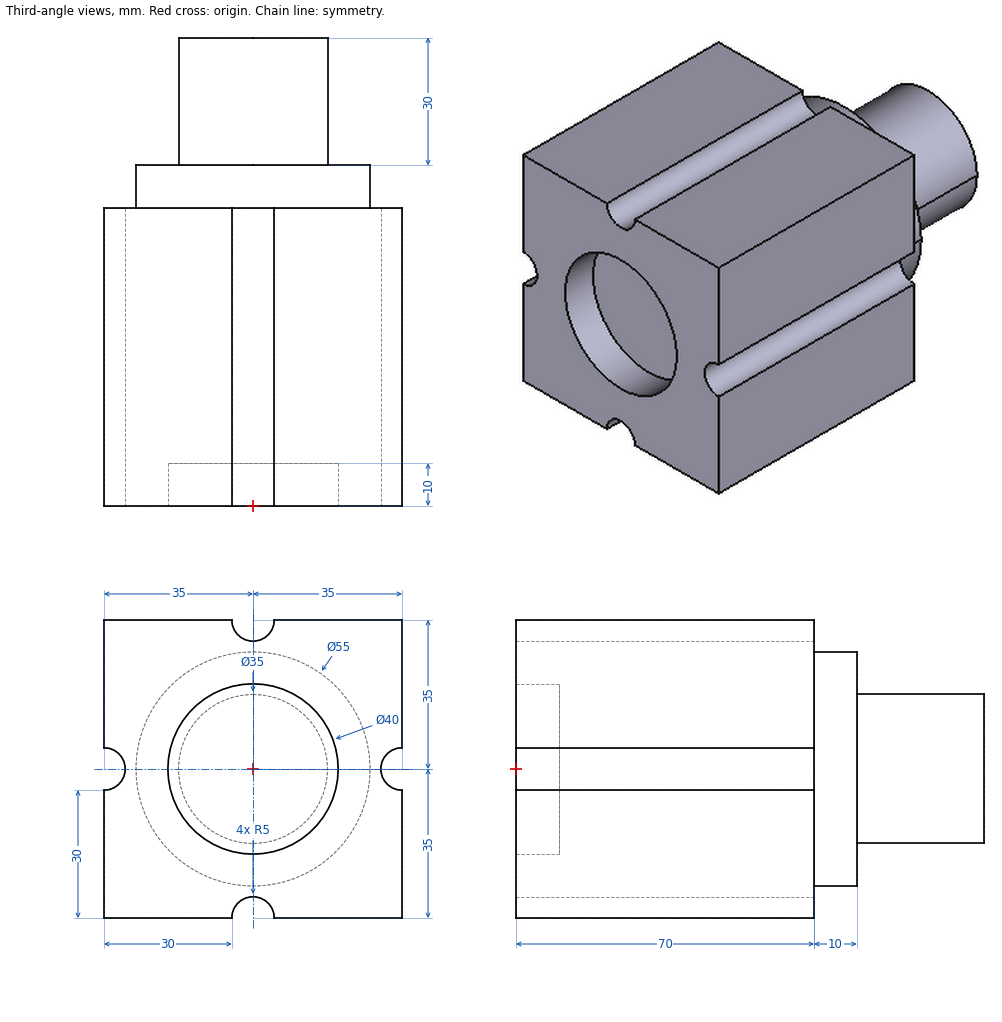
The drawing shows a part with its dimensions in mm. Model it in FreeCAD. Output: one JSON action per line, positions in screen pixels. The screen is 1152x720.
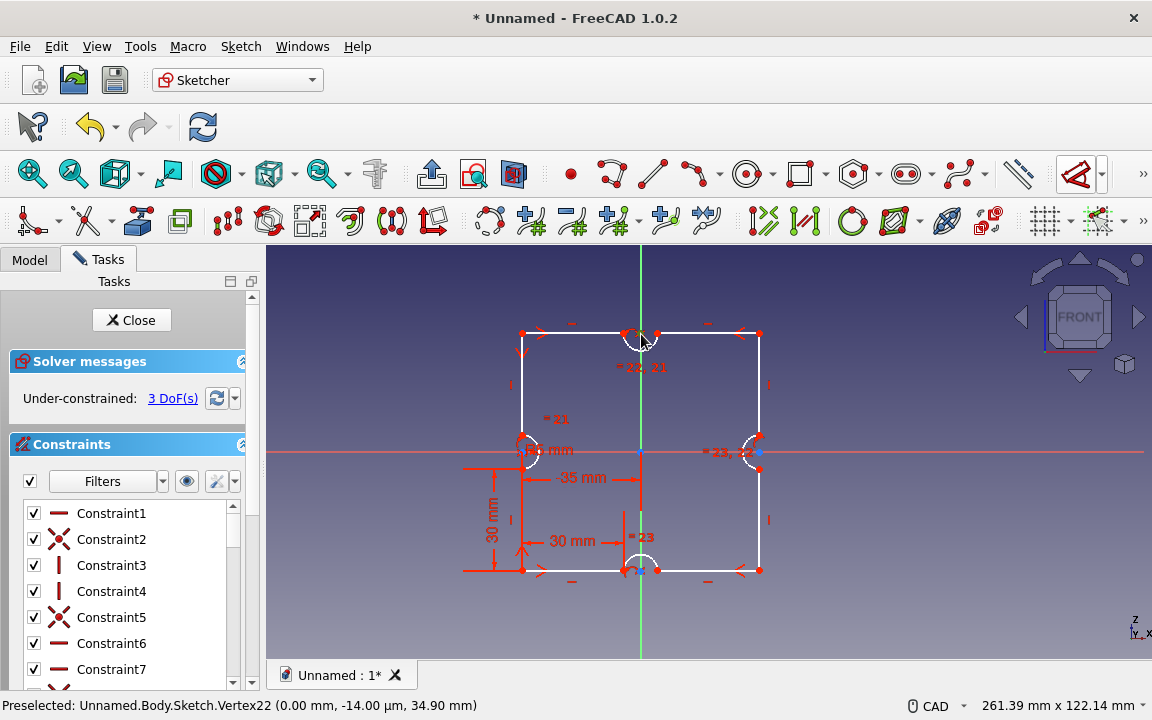
{"action": "key", "text": "i"}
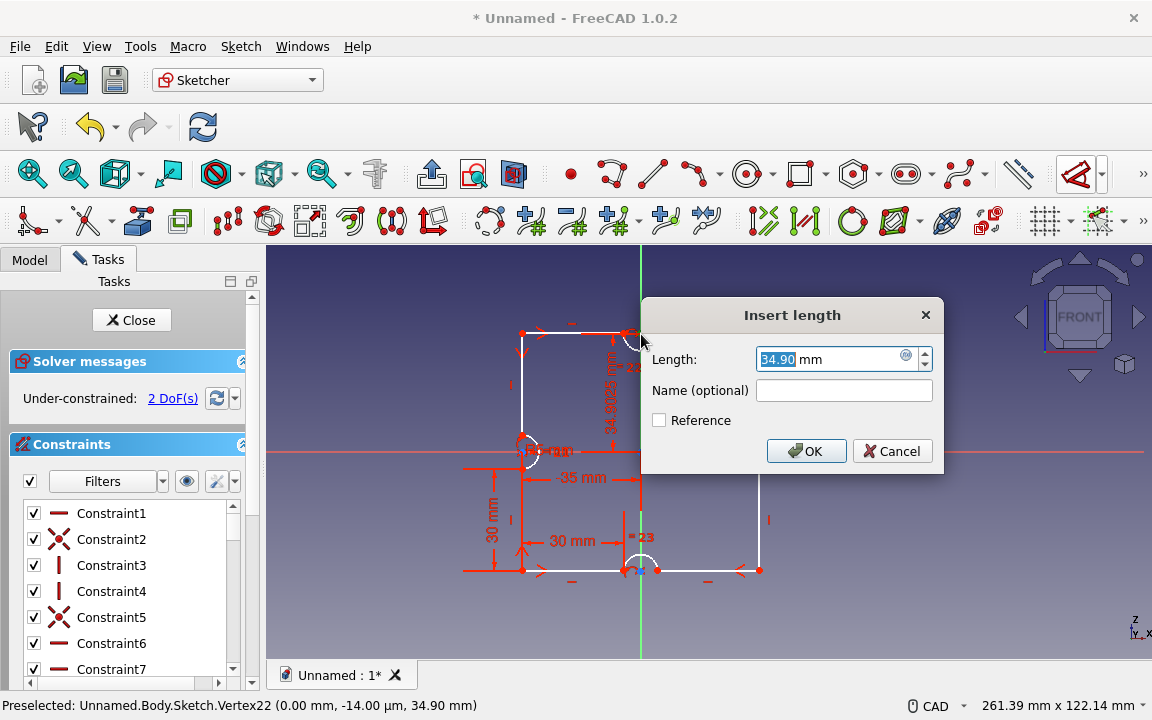
{"action": "type", "text": "35"}
{"action": "key", "text": "Return"}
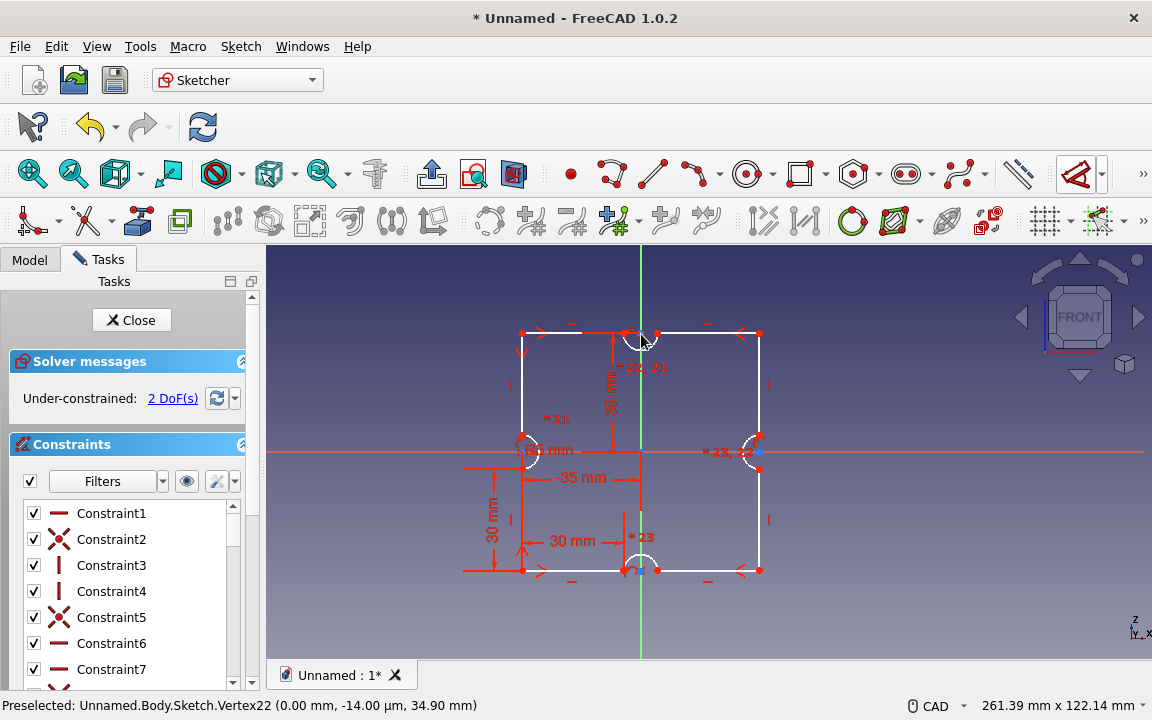
{"action": "left_click", "coordinate": [760, 452]}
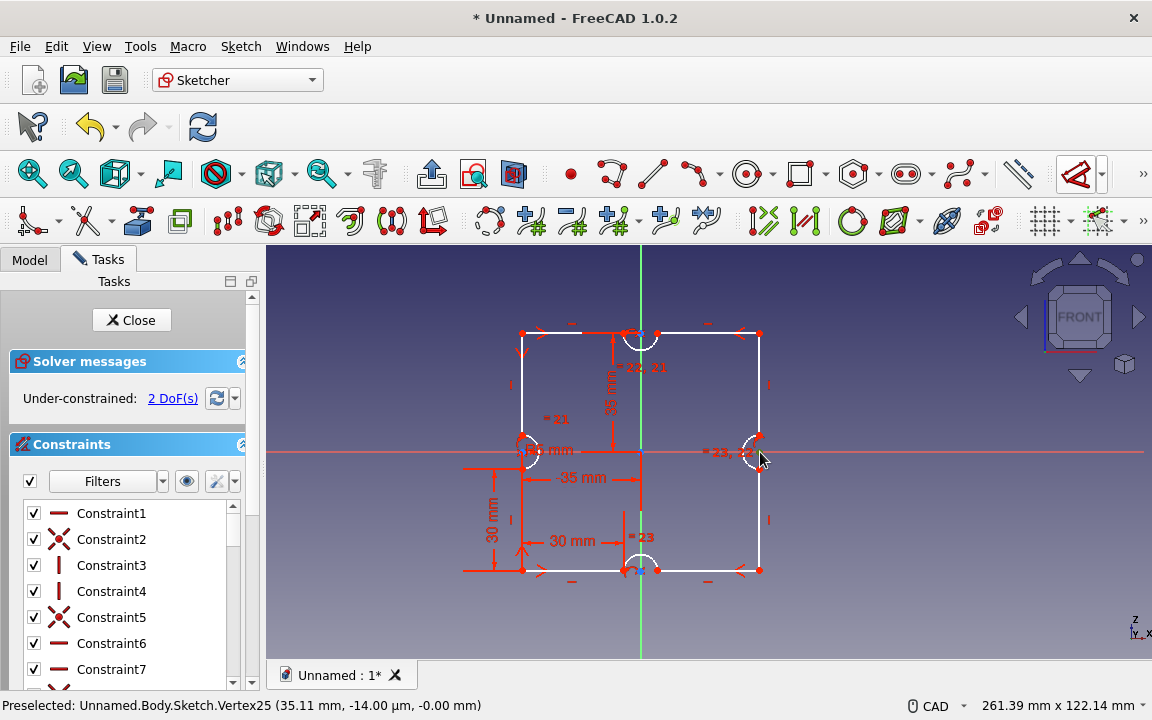
{"action": "key", "text": "l"}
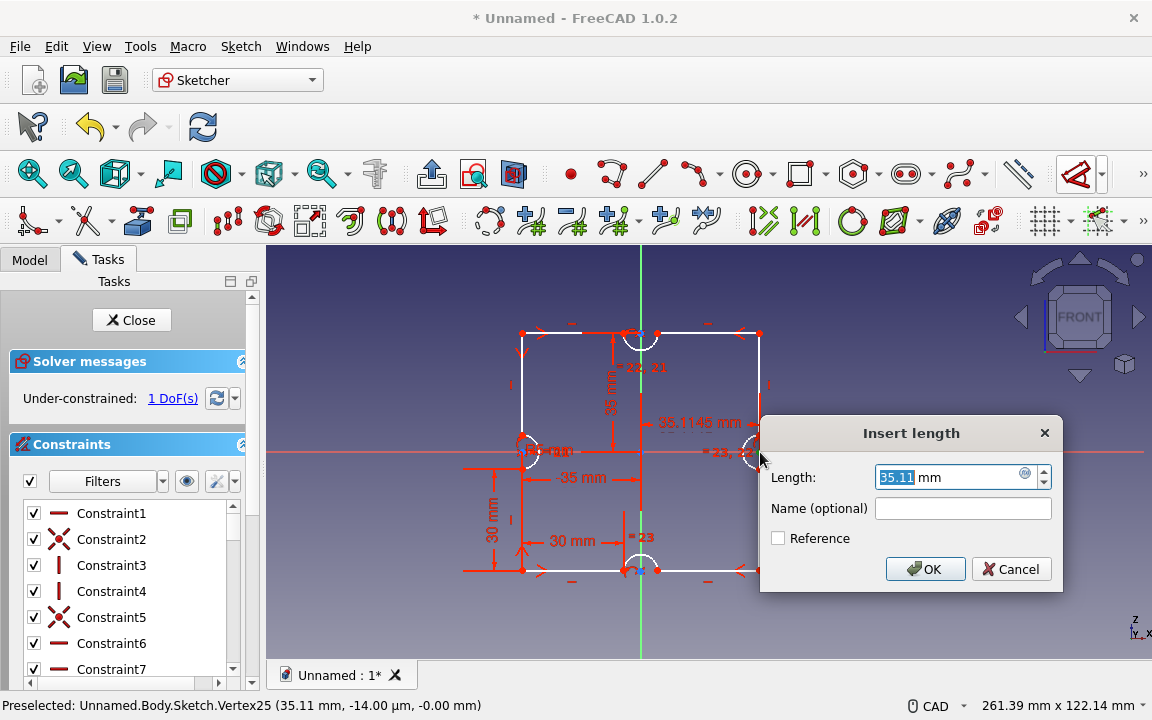
{"action": "type", "text": "35"}
{"action": "key", "text": "Return"}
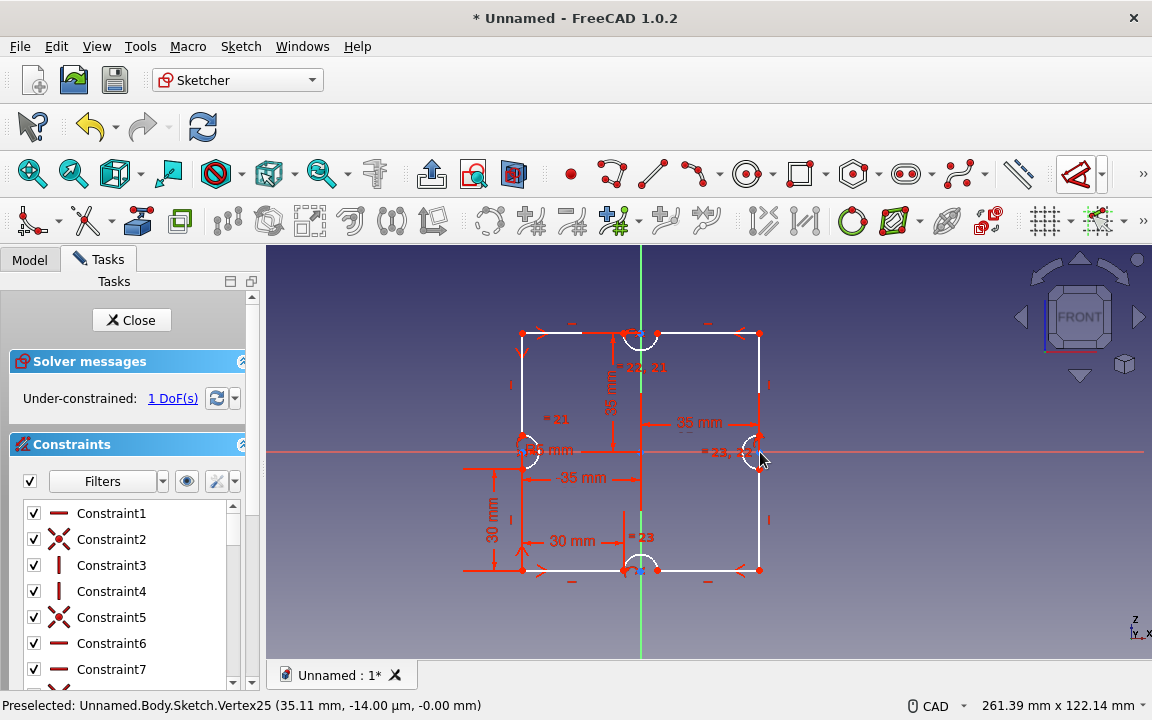
{"action": "left_click", "coordinate": [641, 571]}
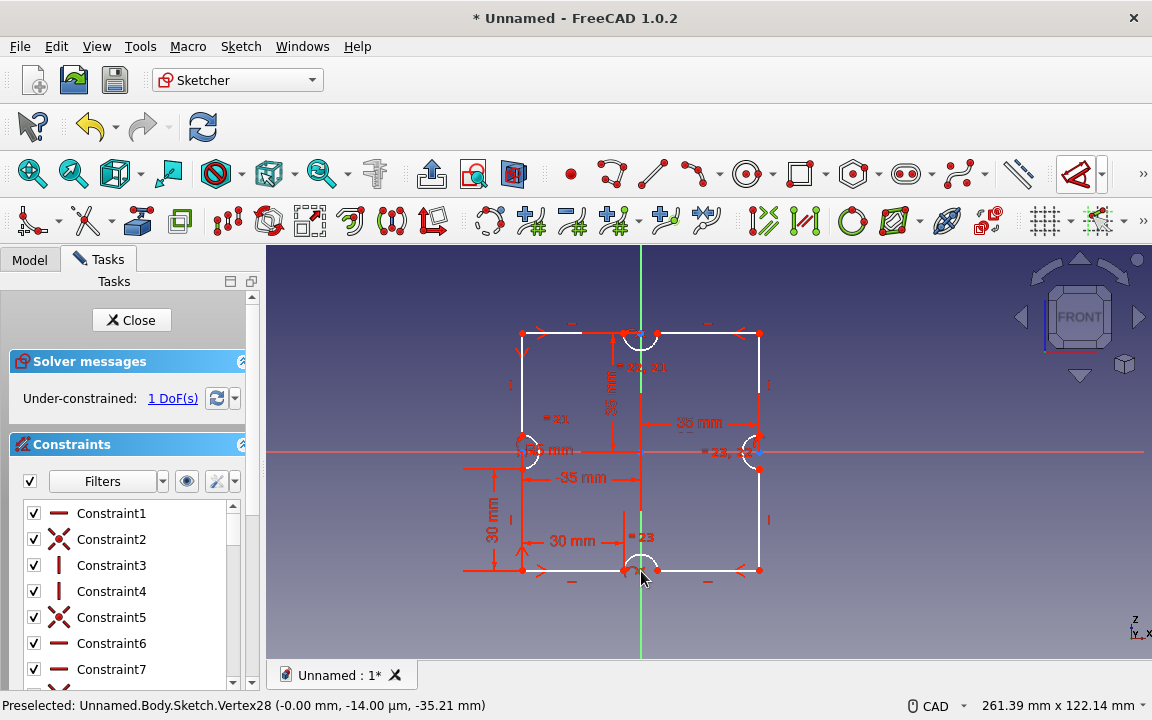
{"action": "left_click", "coordinate": [1102, 174]}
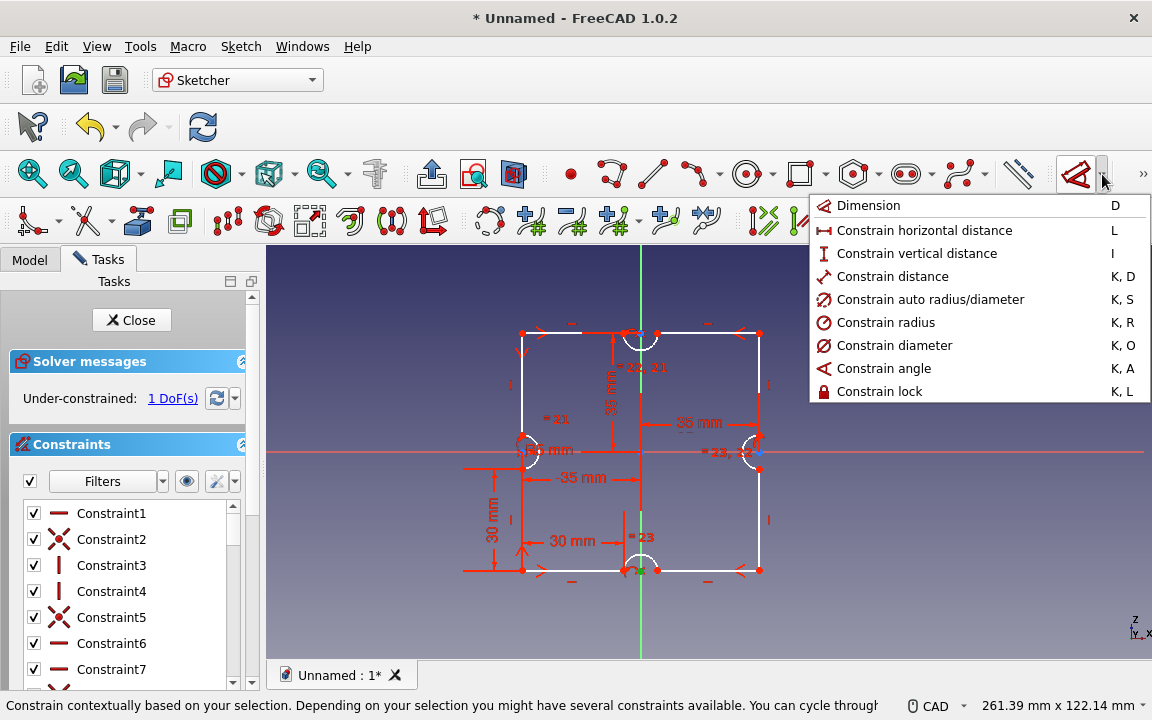
{"action": "left_click", "coordinate": [980, 254]}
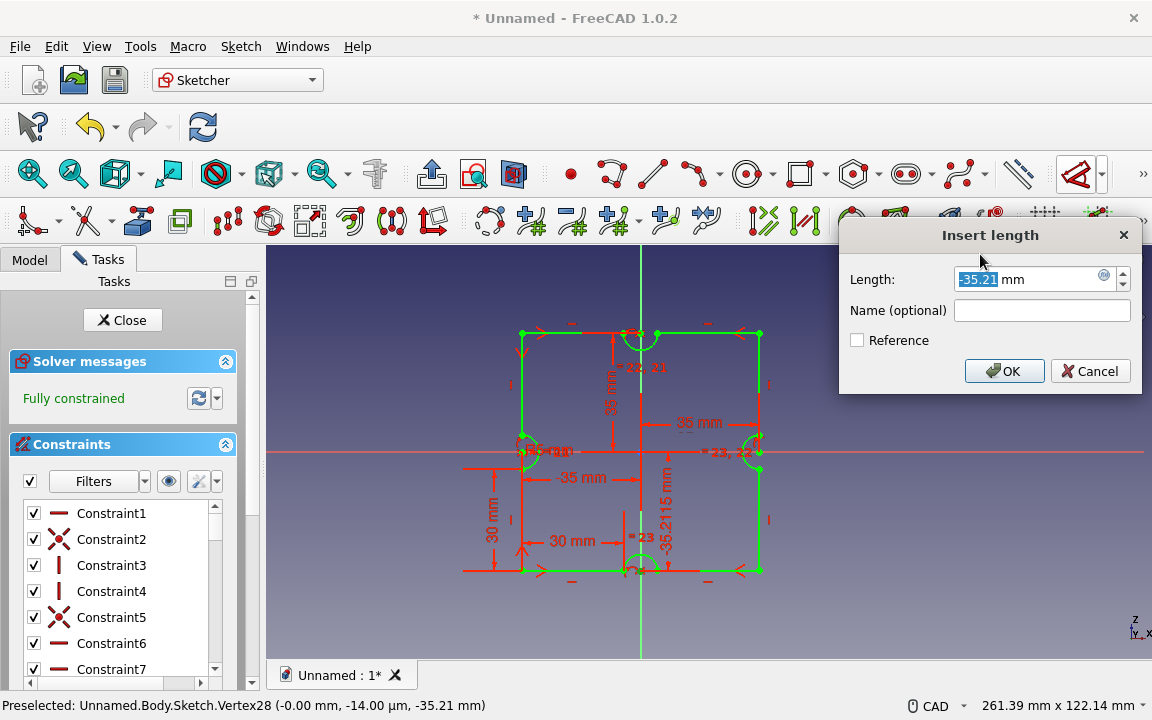
{"action": "type", "text": "-35"}
{"action": "key", "text": "Return"}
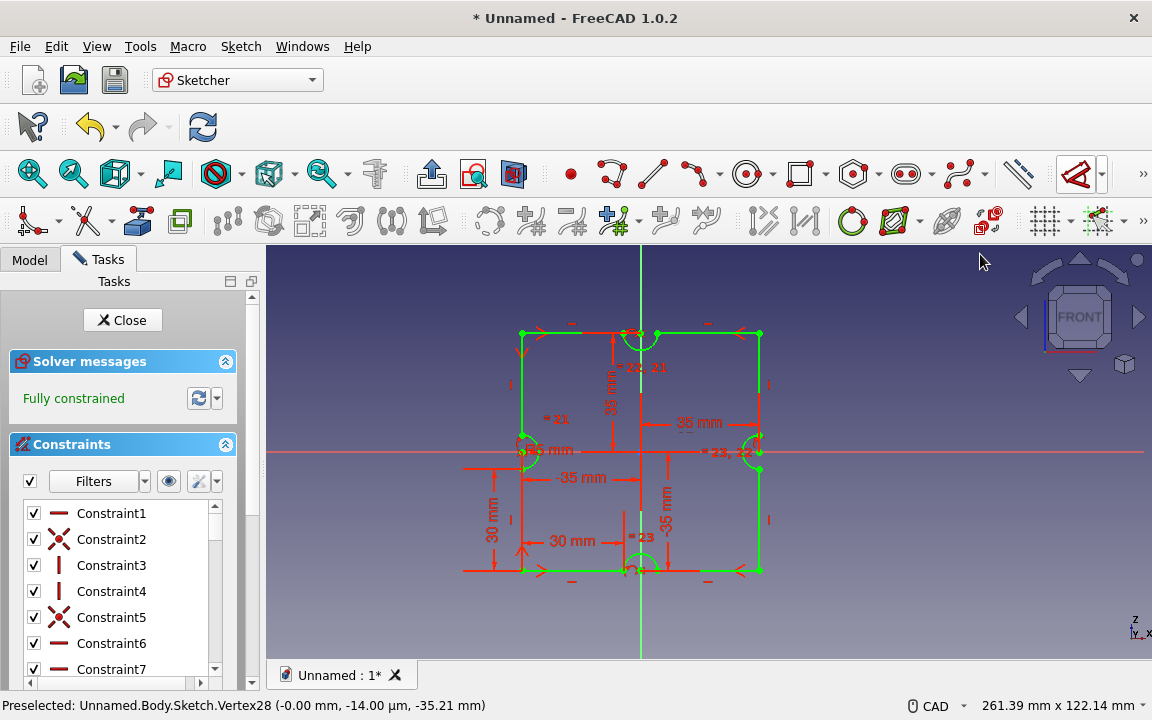
{"action": "left_click", "coordinate": [123, 320]}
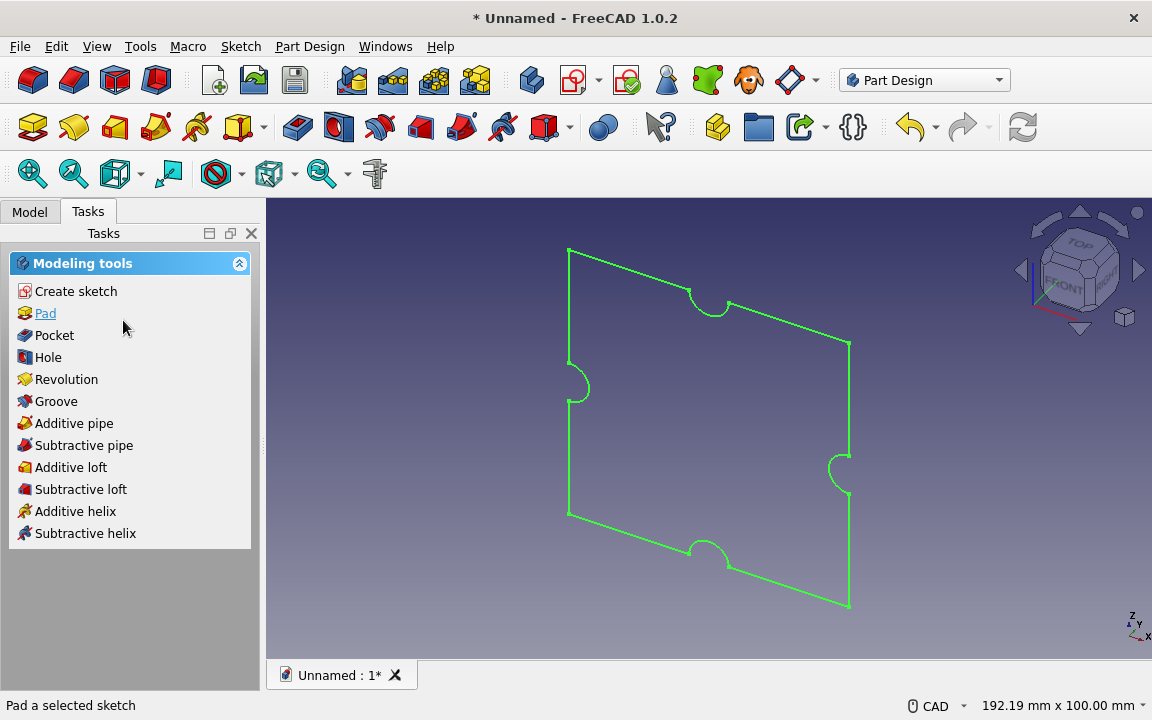
{"action": "left_click", "coordinate": [33, 128]}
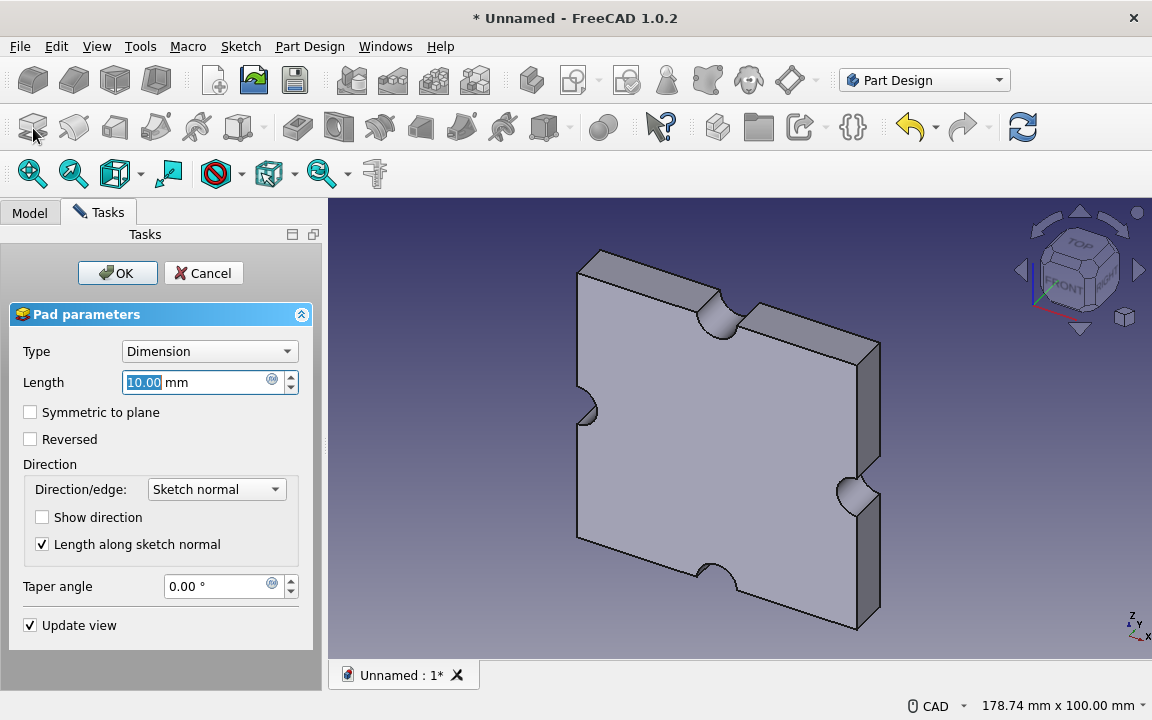
{"action": "type", "text": "70"}
{"action": "key", "text": "Tab"}